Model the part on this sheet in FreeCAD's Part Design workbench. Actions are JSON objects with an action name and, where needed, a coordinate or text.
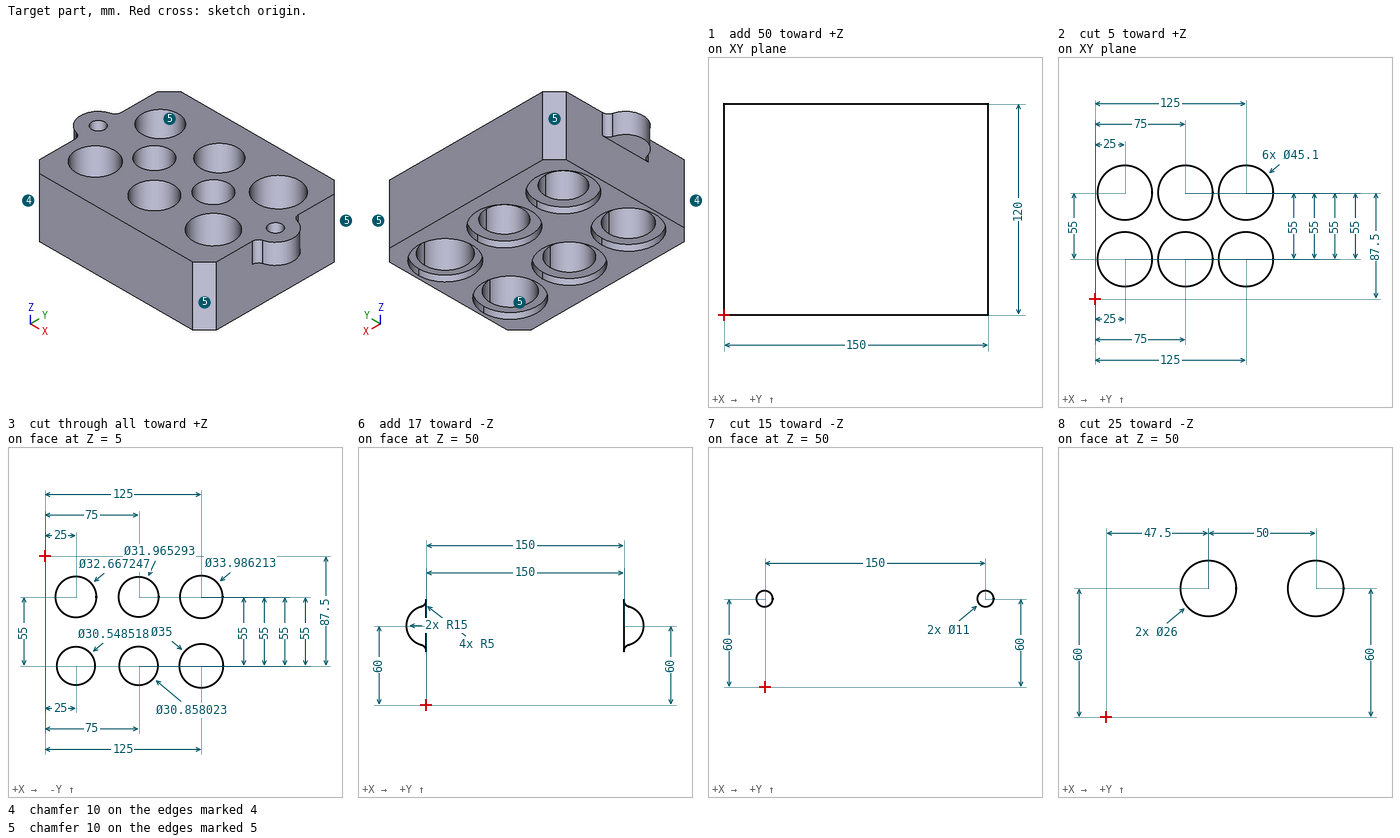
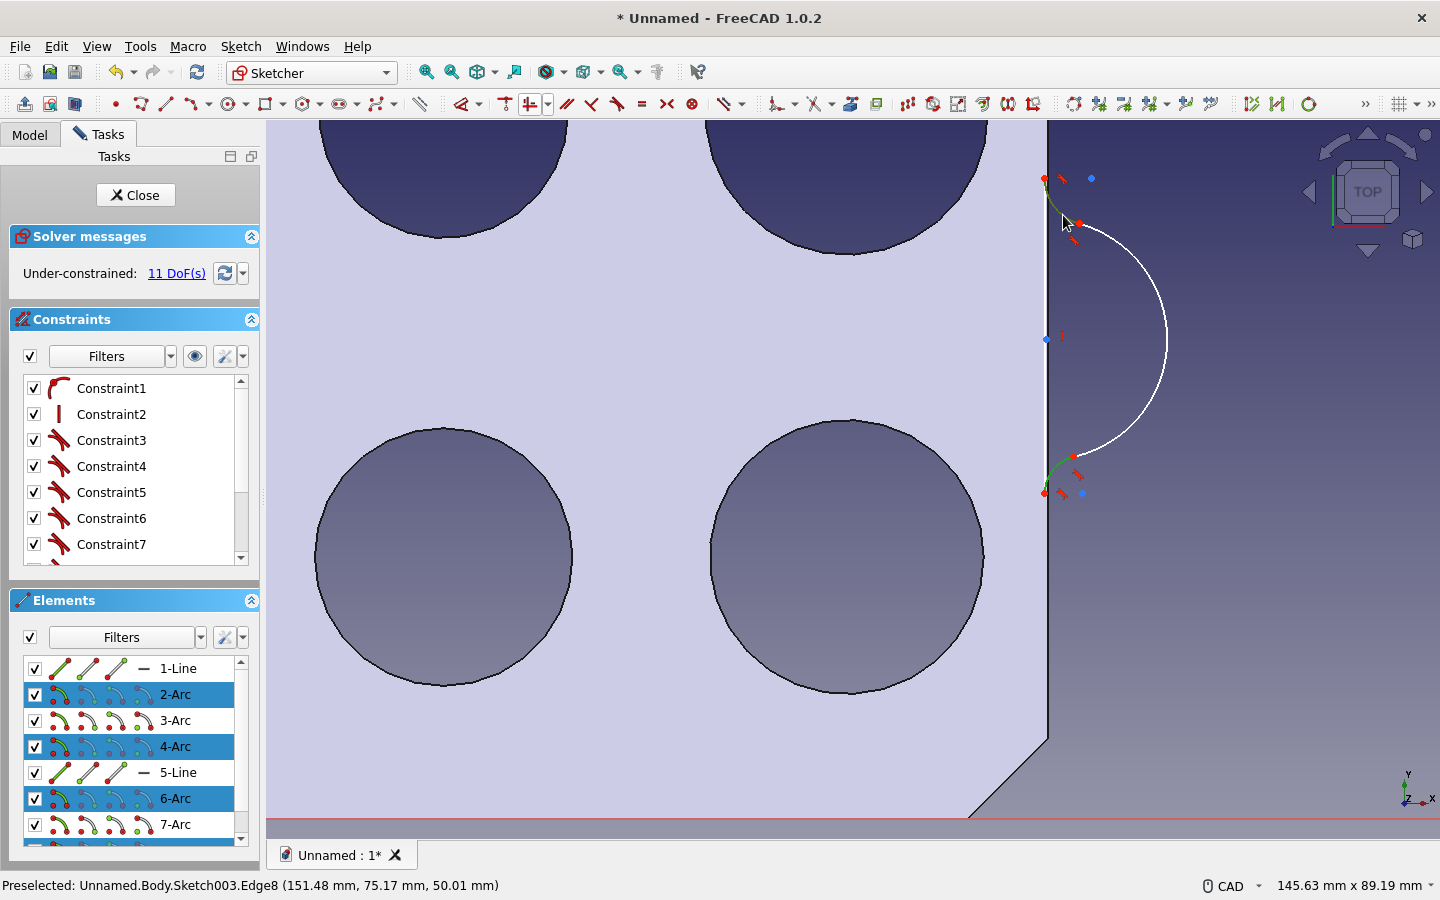
{"action": "left_click", "coordinate": [642, 104]}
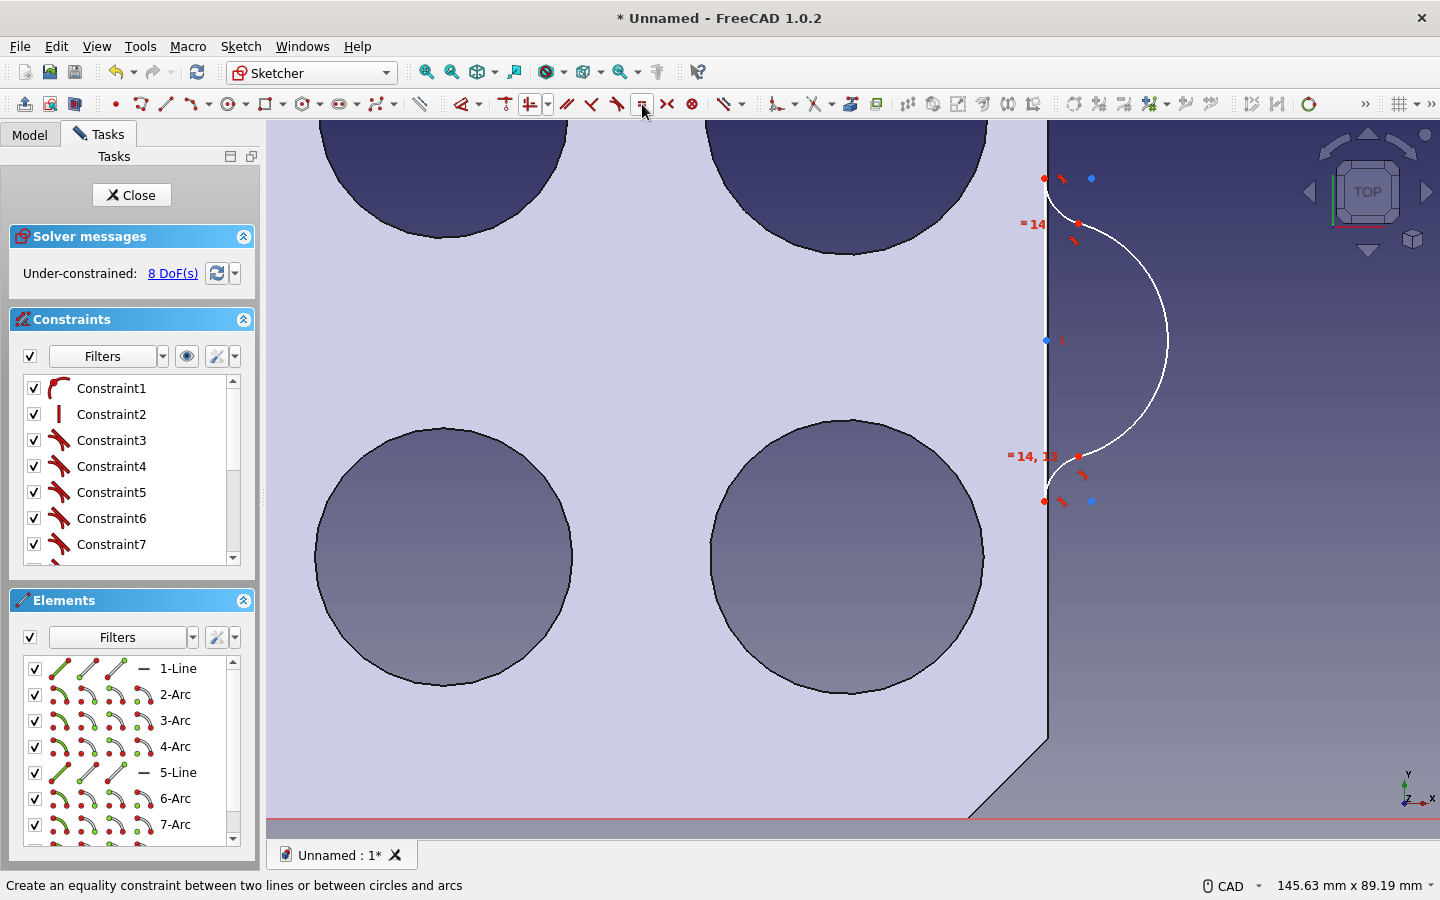
{"action": "scroll", "coordinate": [1063, 463], "scroll_direction": "down", "scroll_amount": 4}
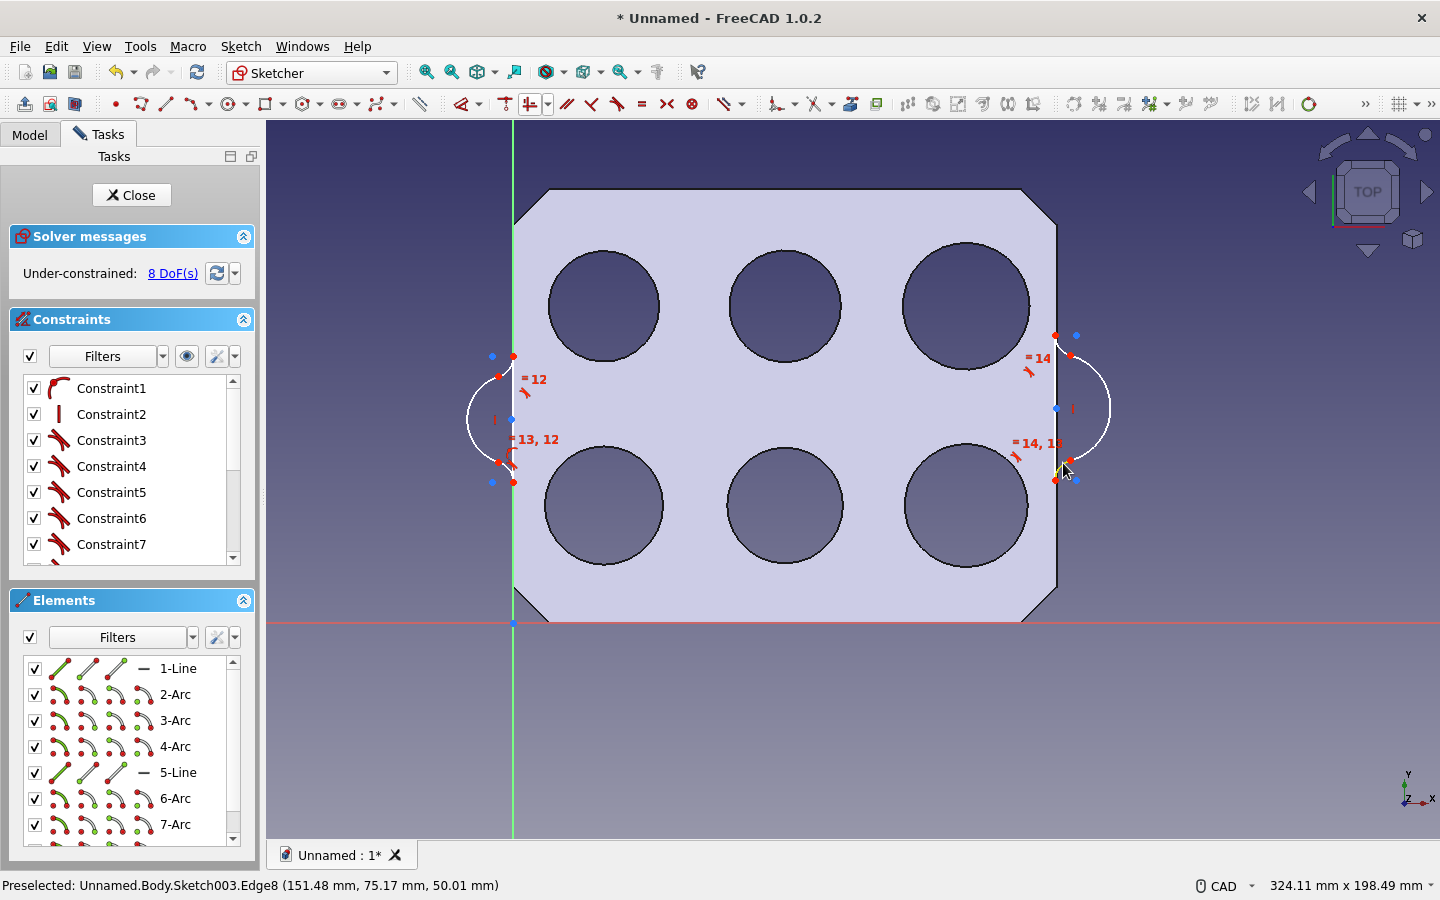
{"action": "left_click", "coordinate": [473, 398]}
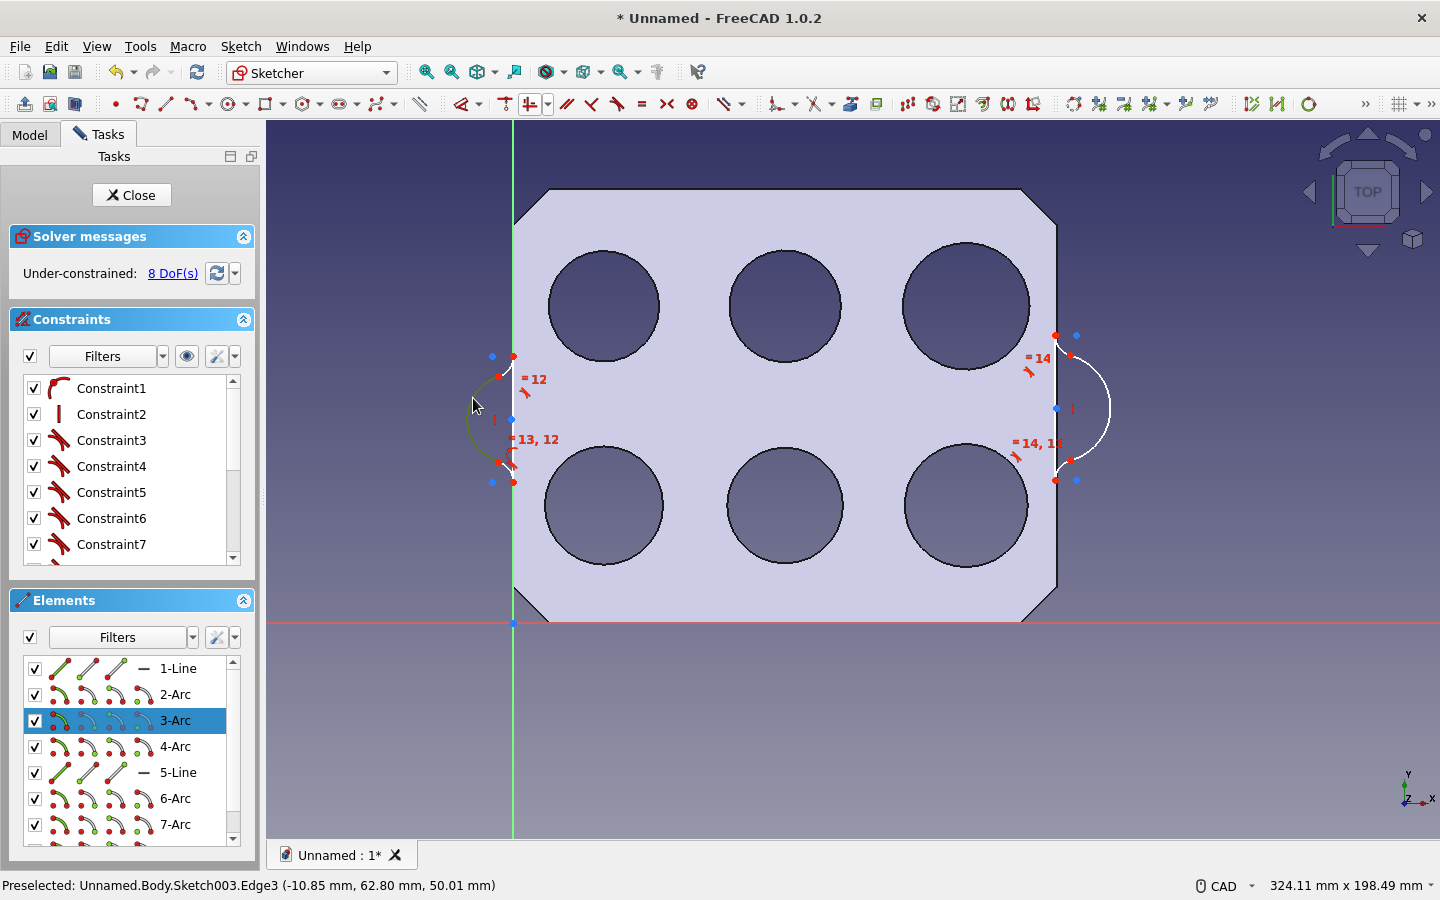
{"action": "left_click", "coordinate": [1103, 435]}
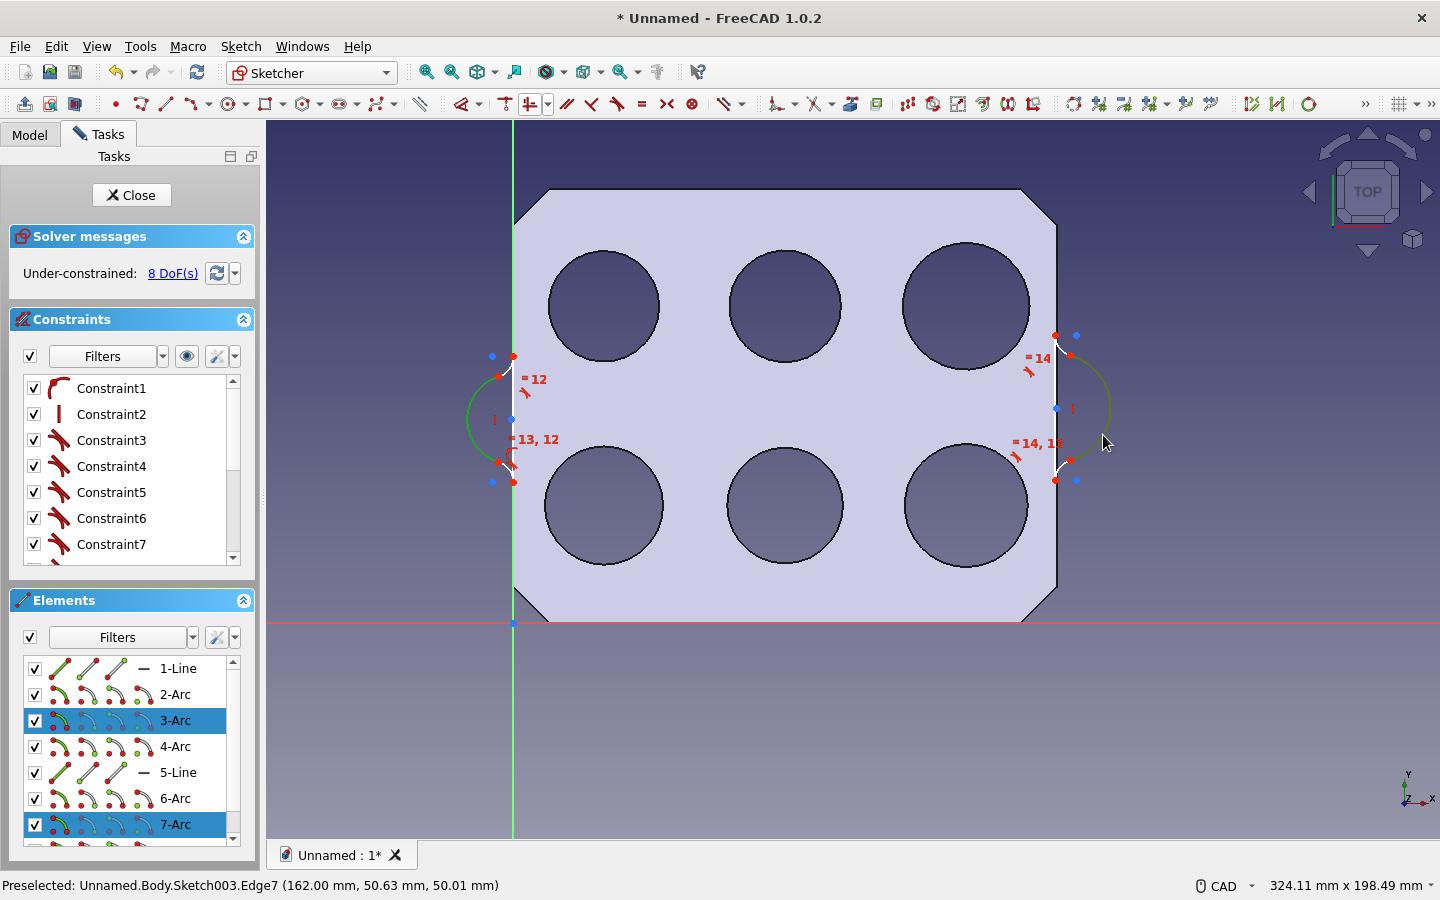
{"action": "left_click", "coordinate": [642, 104]}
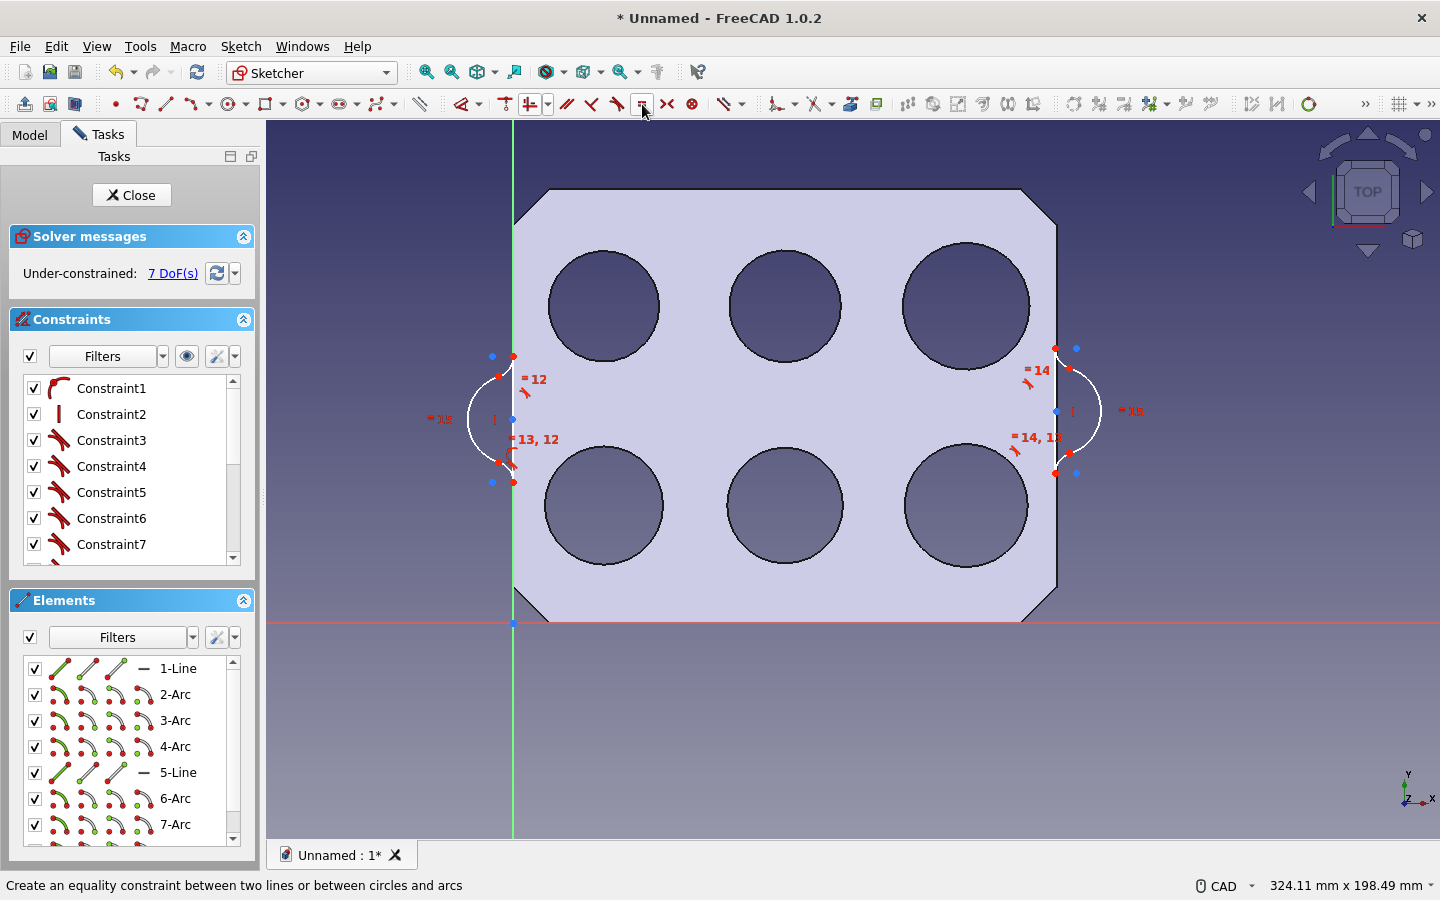
{"action": "left_click", "coordinate": [512, 419]}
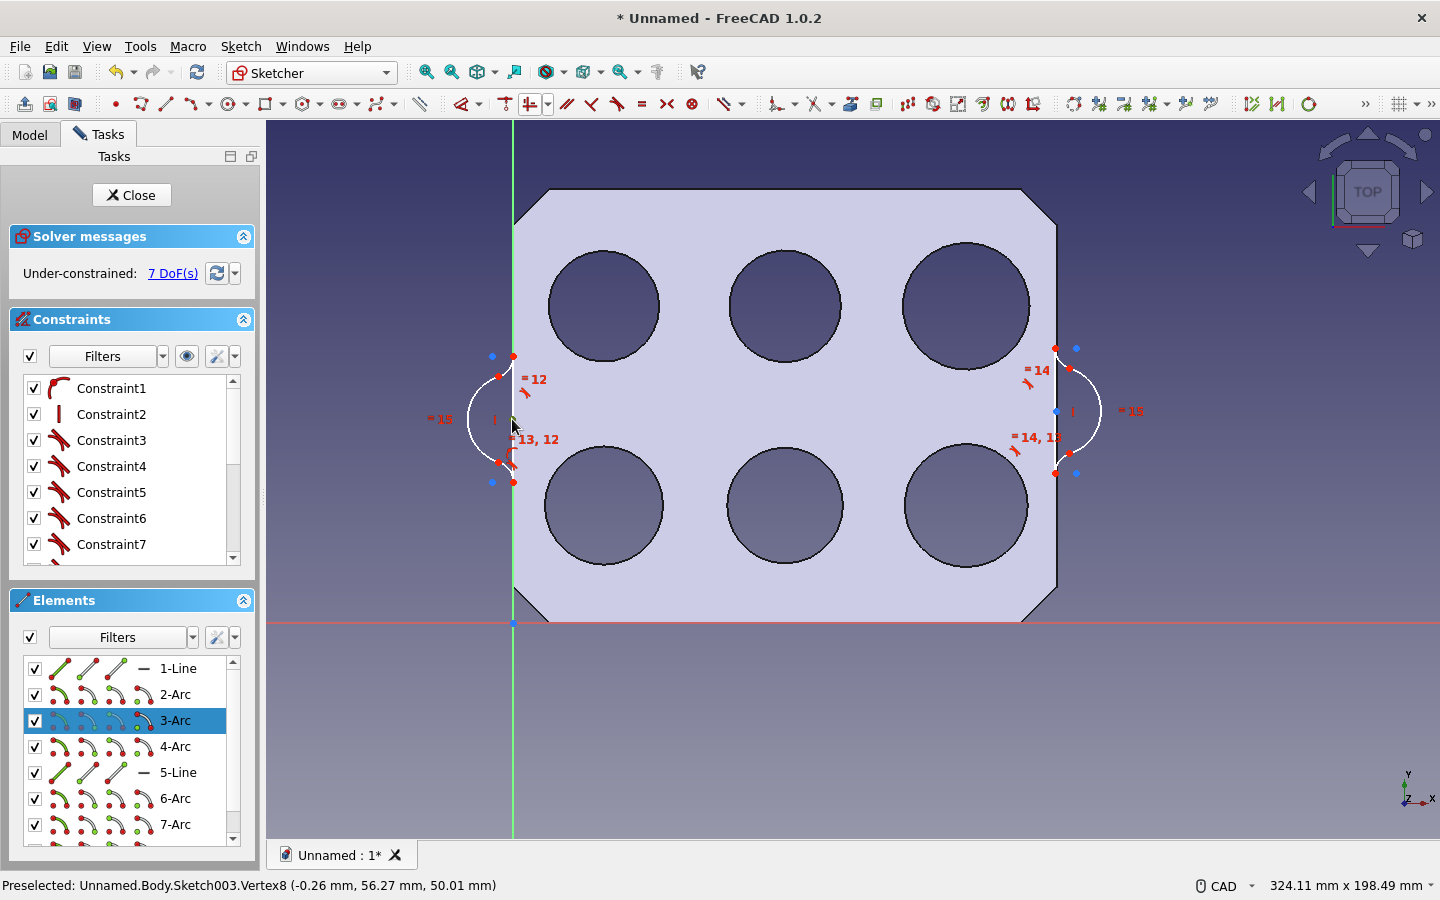
{"action": "left_click", "coordinate": [513, 764]}